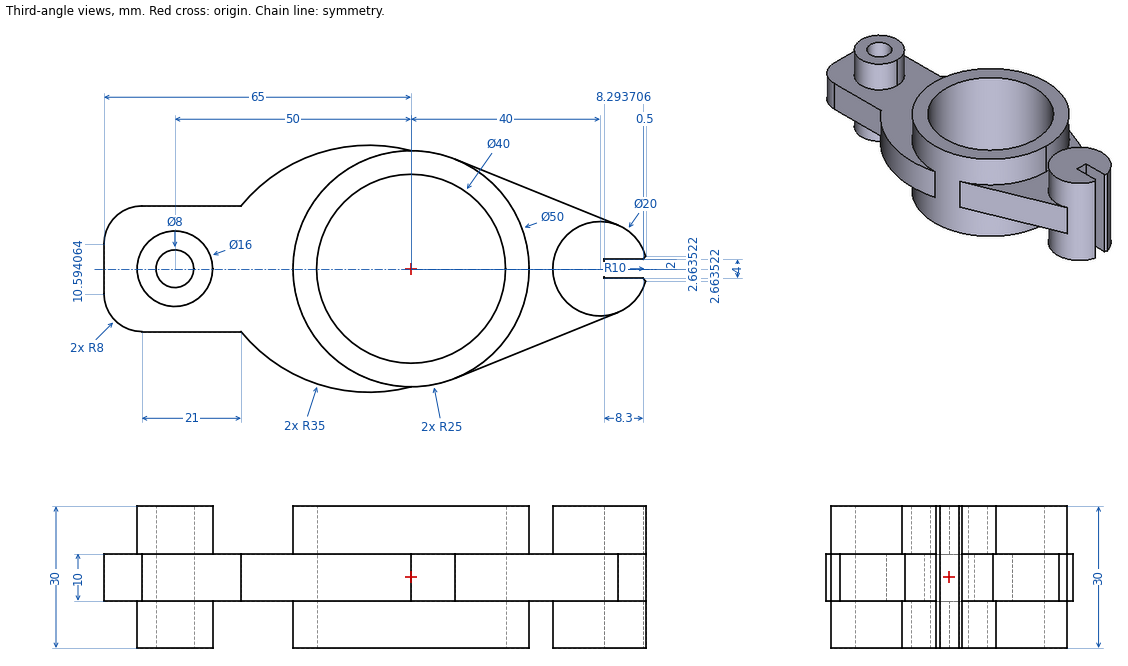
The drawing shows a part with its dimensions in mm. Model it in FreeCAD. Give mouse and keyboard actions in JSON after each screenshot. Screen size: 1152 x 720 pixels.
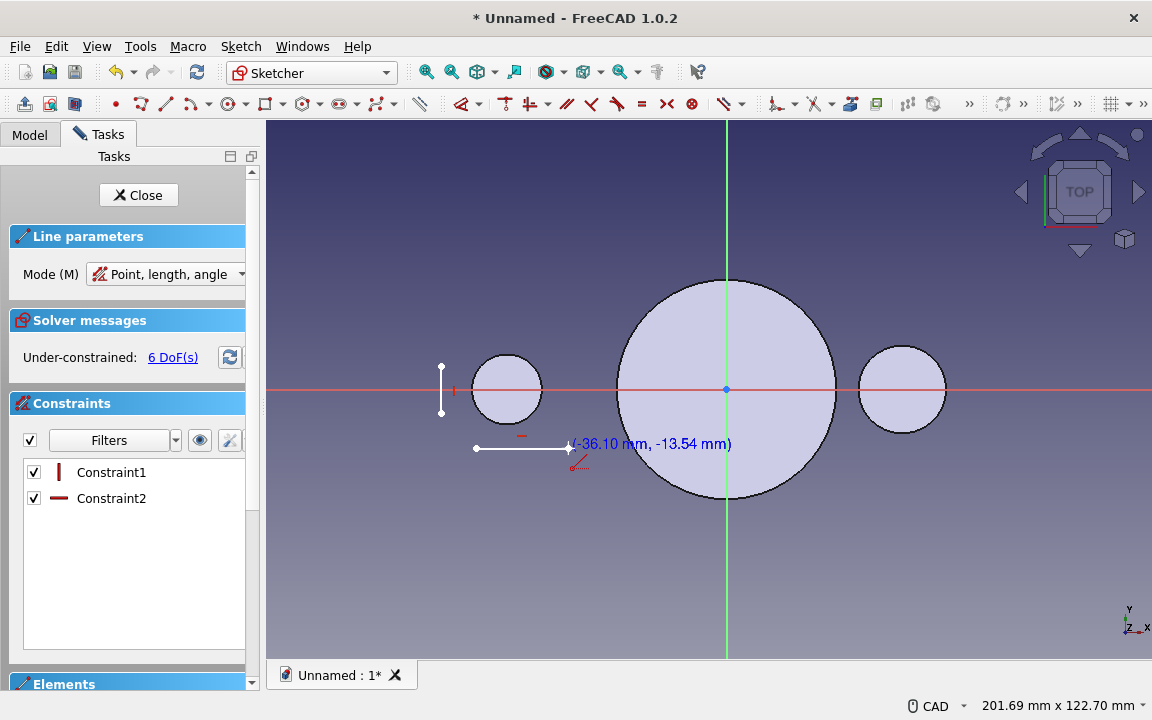
{"action": "left_click", "coordinate": [768, 491]}
{"action": "left_click", "coordinate": [919, 430]}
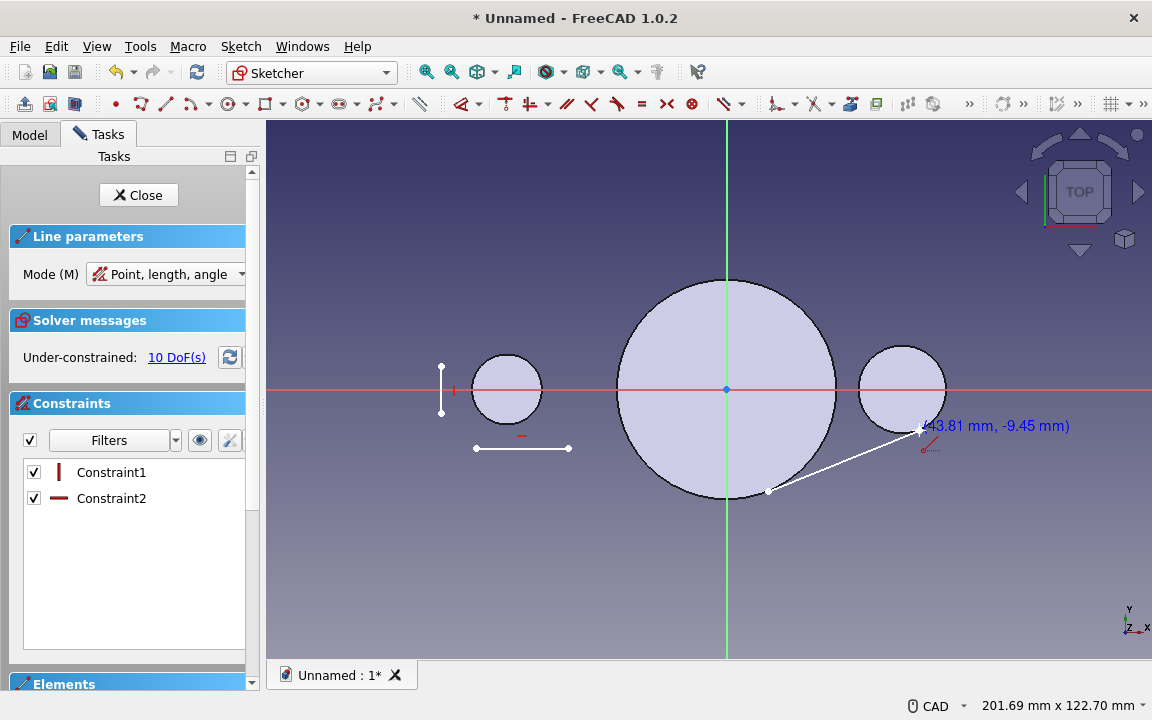
{"action": "left_click", "coordinate": [919, 349]}
{"action": "left_click", "coordinate": [768, 288]}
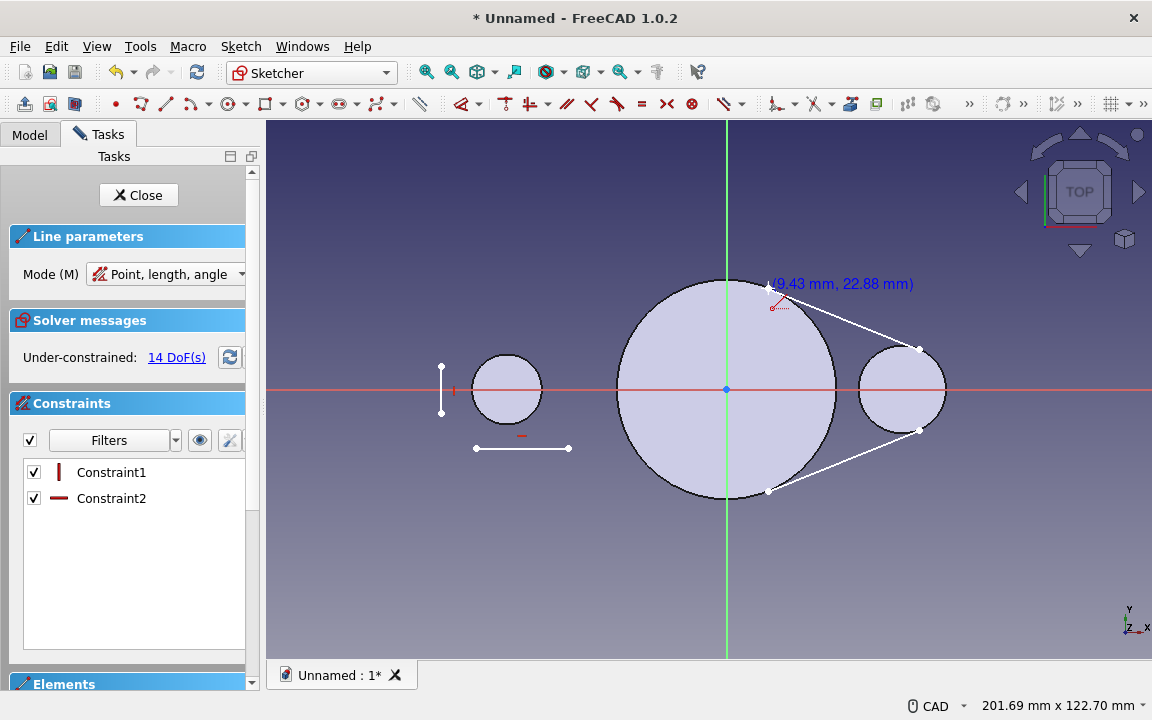
{"action": "left_click", "coordinate": [568, 331]}
{"action": "left_click", "coordinate": [476, 331]}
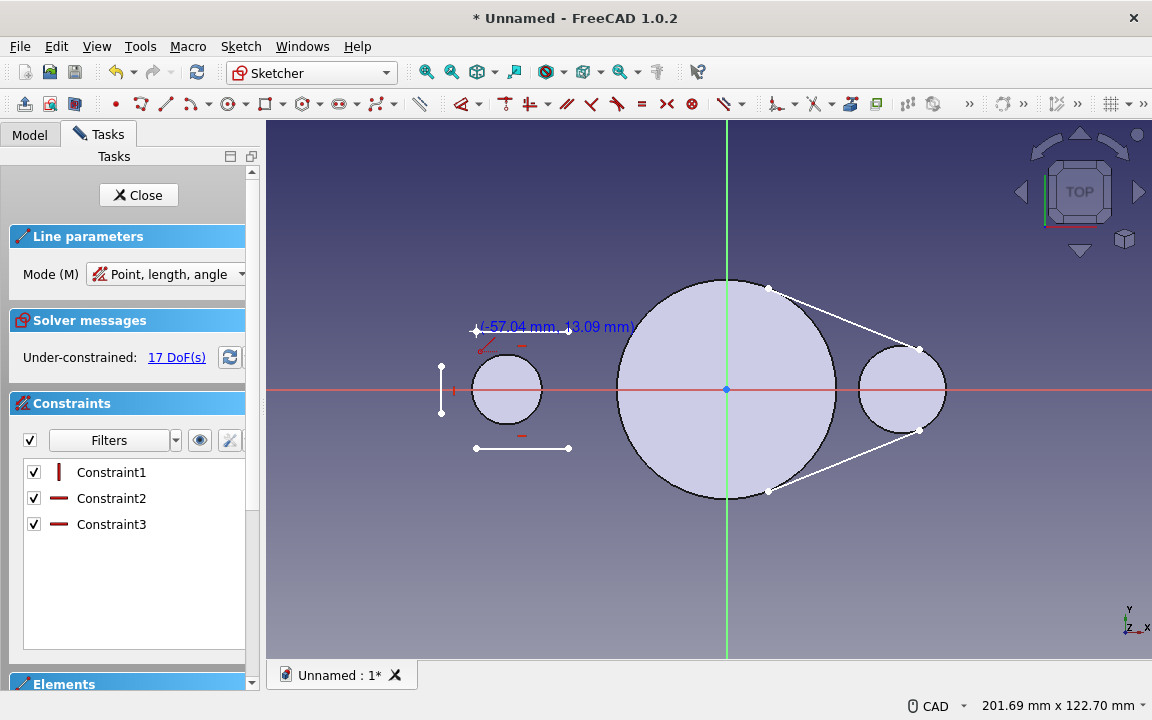
{"action": "key", "text": "g 3 a"}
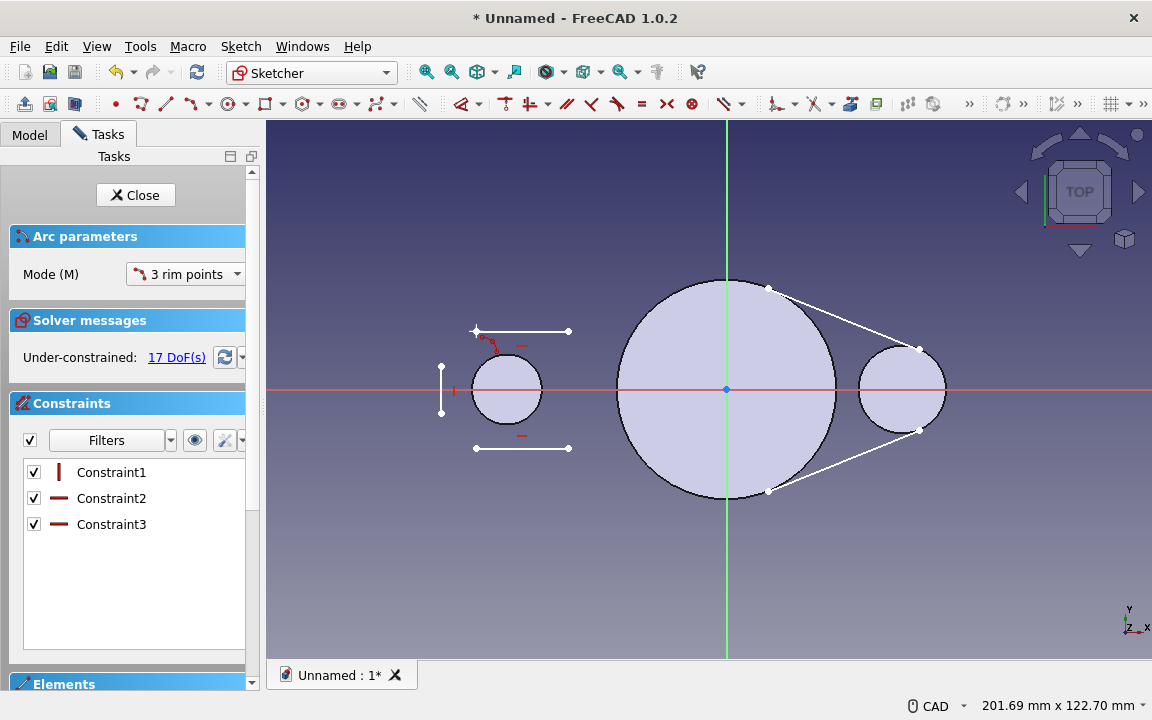
{"action": "left_click", "coordinate": [441, 414]}
{"action": "left_click", "coordinate": [476, 449]}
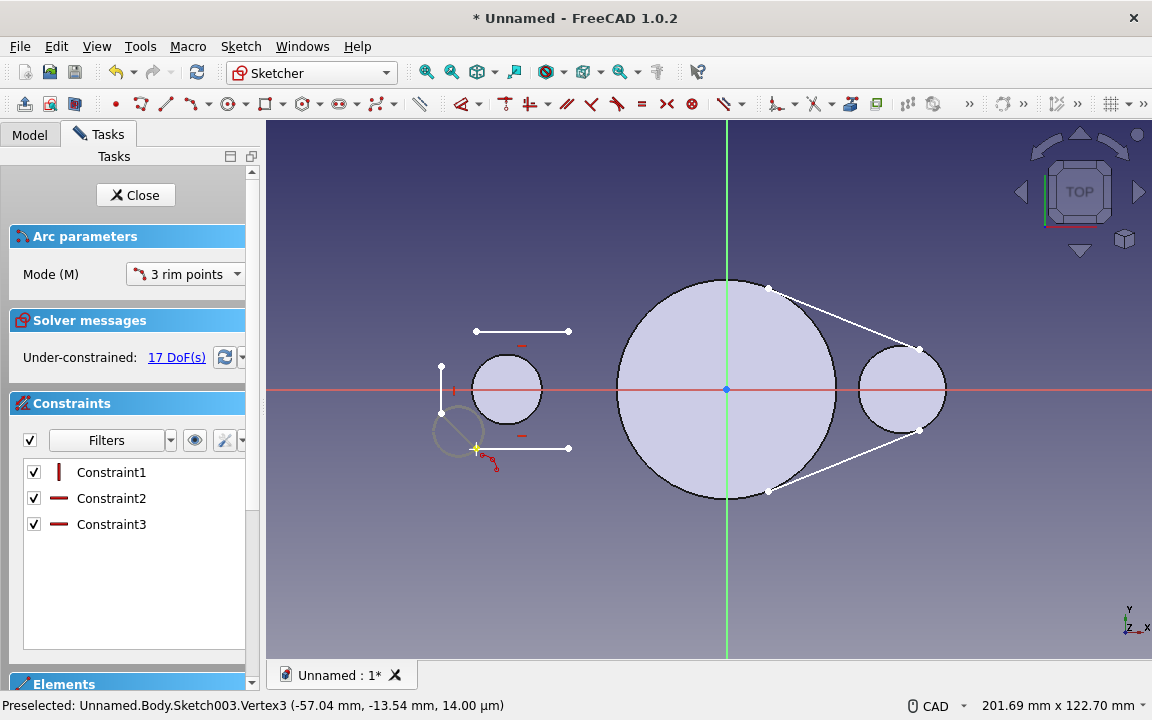
{"action": "scroll", "coordinate": [451, 438], "scroll_direction": "up", "scroll_amount": 3}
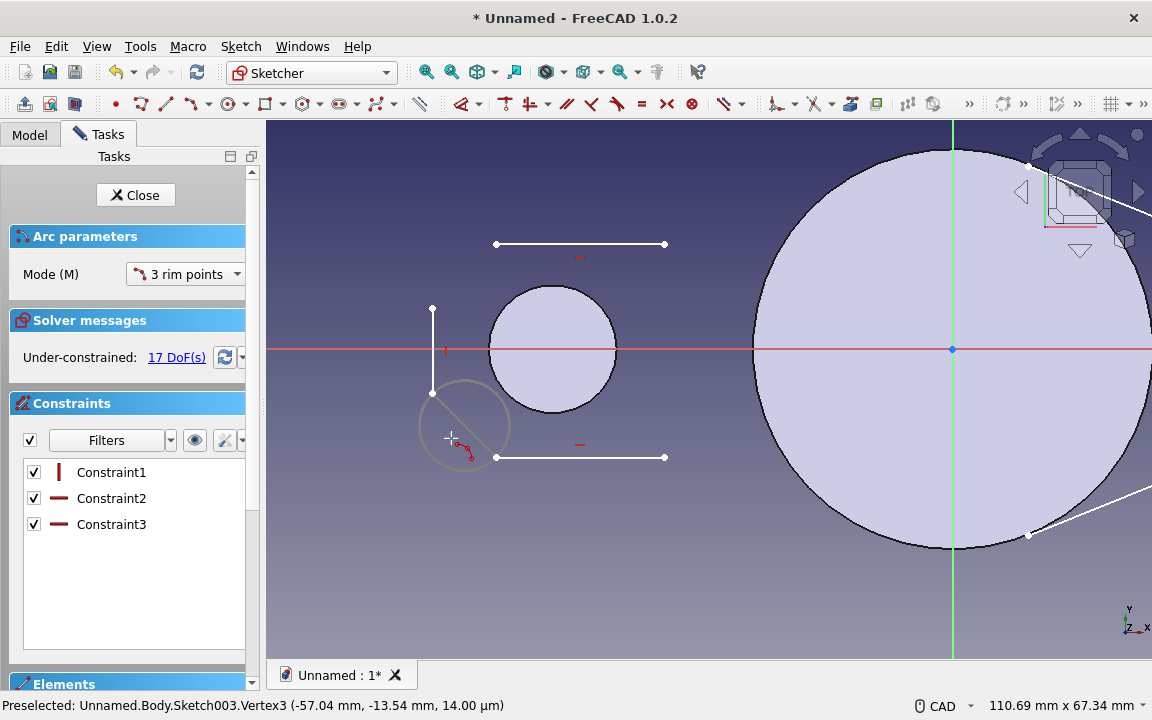
{"action": "left_click", "coordinate": [451, 437]}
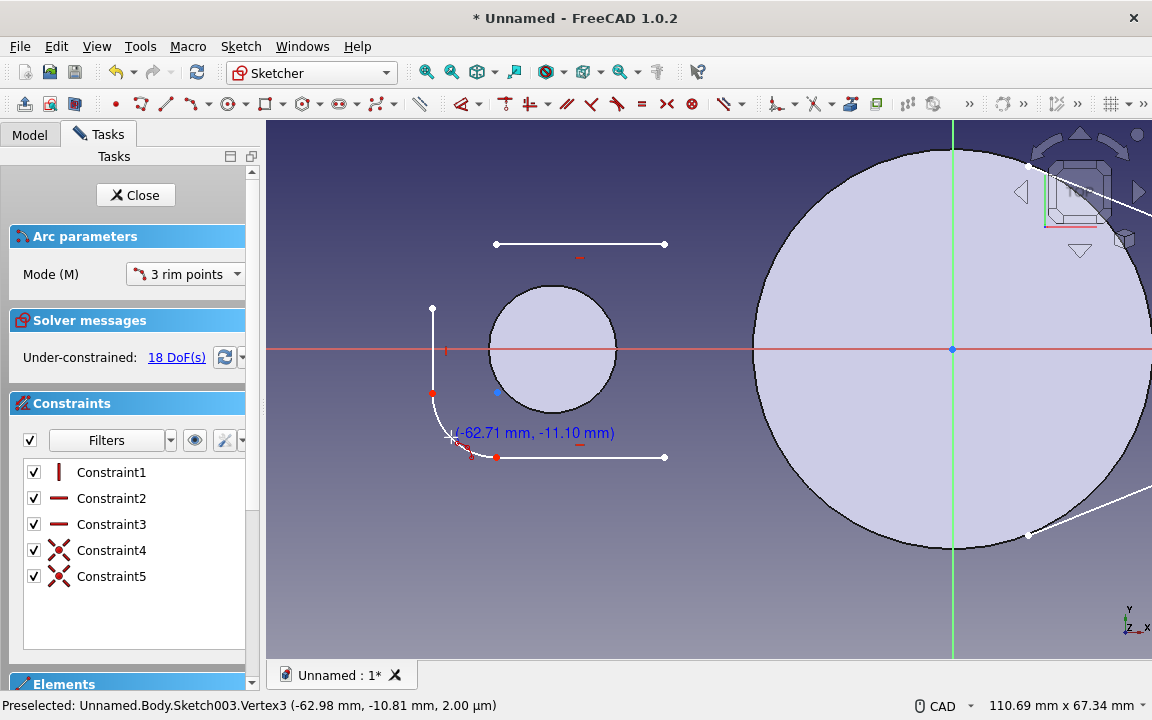
{"action": "left_click", "coordinate": [664, 458]}
{"action": "left_click", "coordinate": [953, 549]}
{"action": "left_click", "coordinate": [795, 545]}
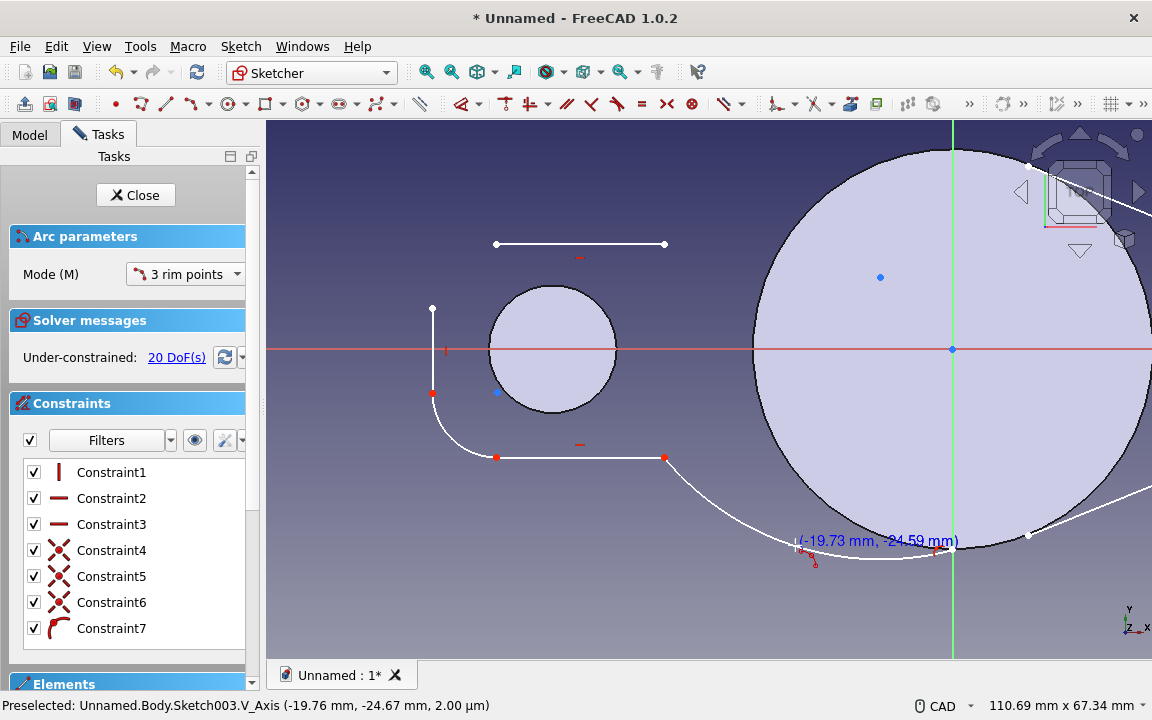
{"action": "left_click", "coordinate": [953, 550]}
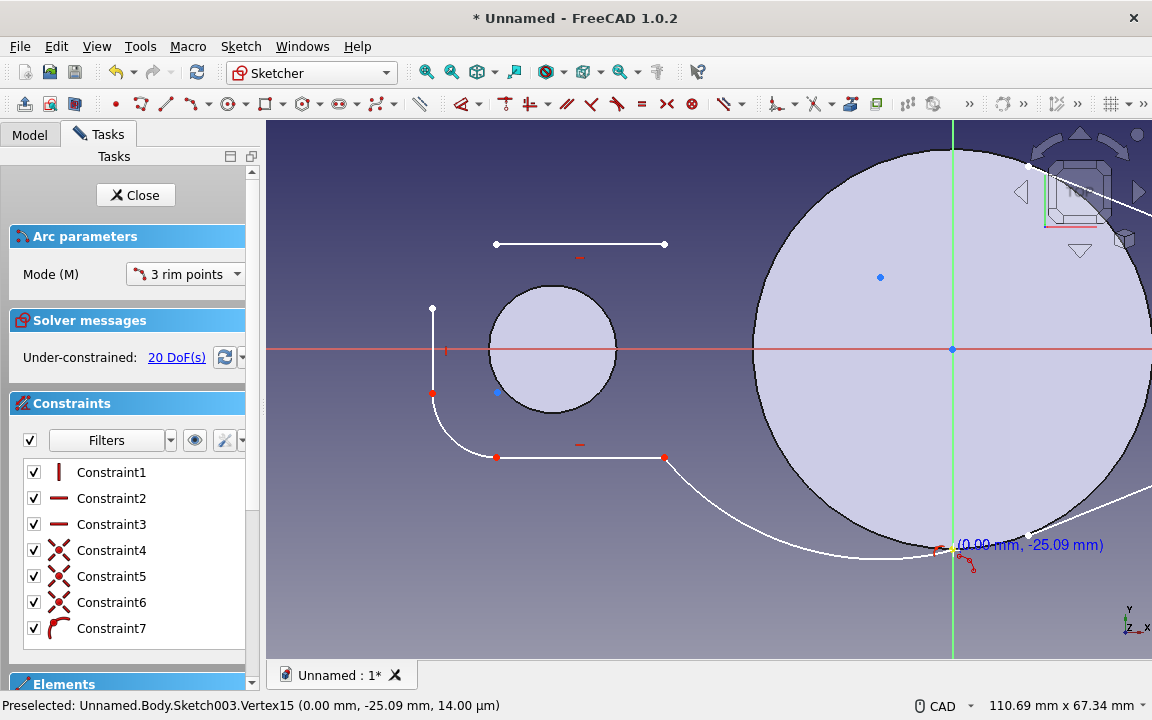
{"action": "scroll", "coordinate": [333, 439], "scroll_direction": "down", "scroll_amount": 3}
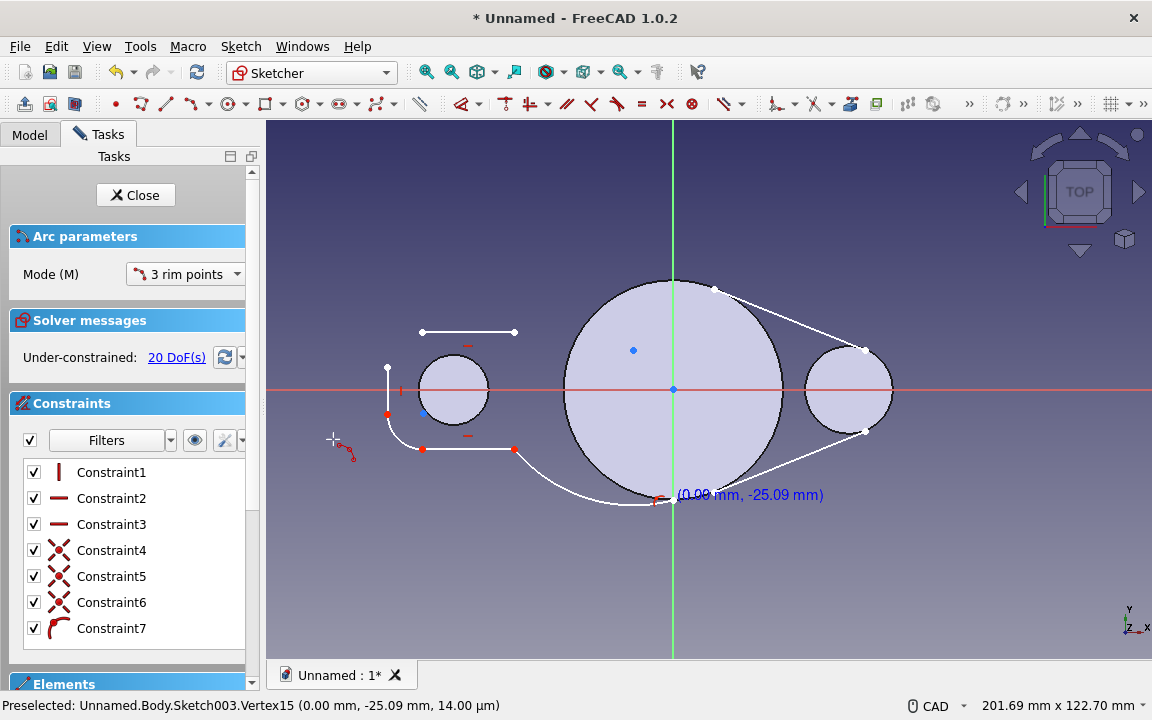
{"action": "left_click", "coordinate": [715, 492]}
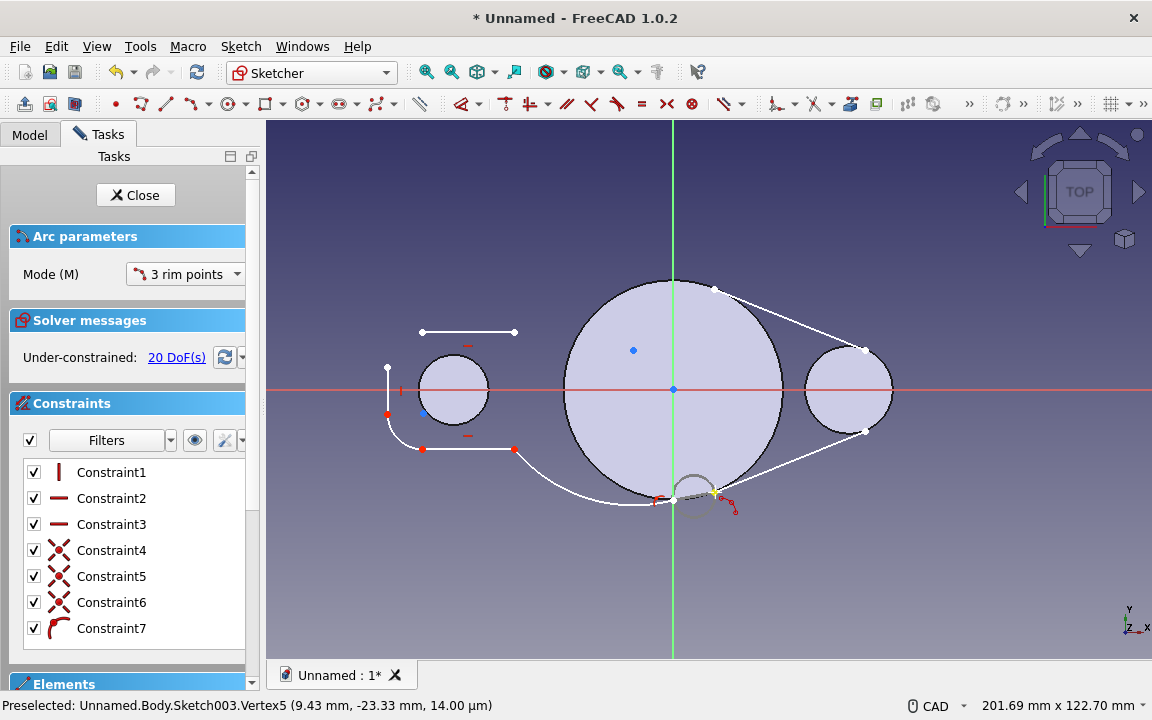
{"action": "scroll", "coordinate": [694, 498], "scroll_direction": "up", "scroll_amount": 11}